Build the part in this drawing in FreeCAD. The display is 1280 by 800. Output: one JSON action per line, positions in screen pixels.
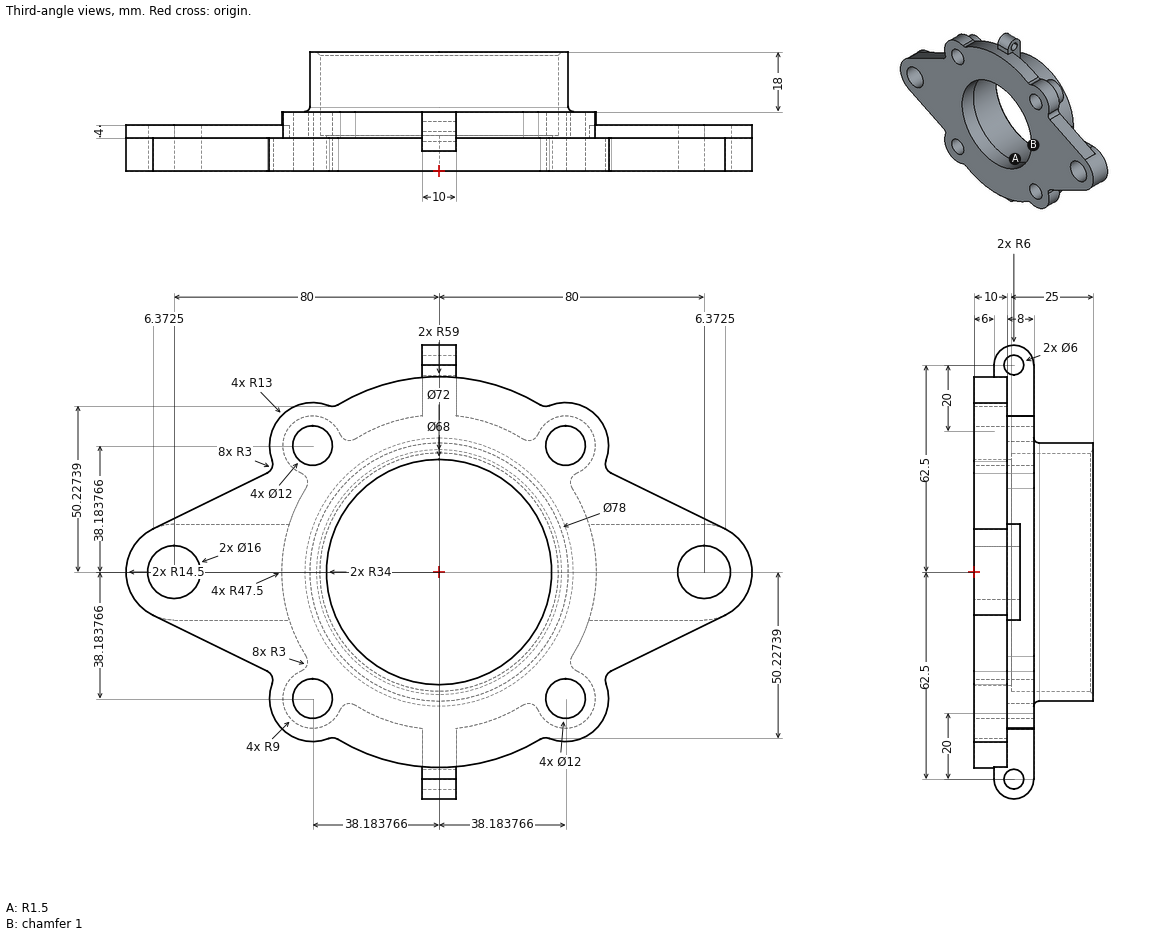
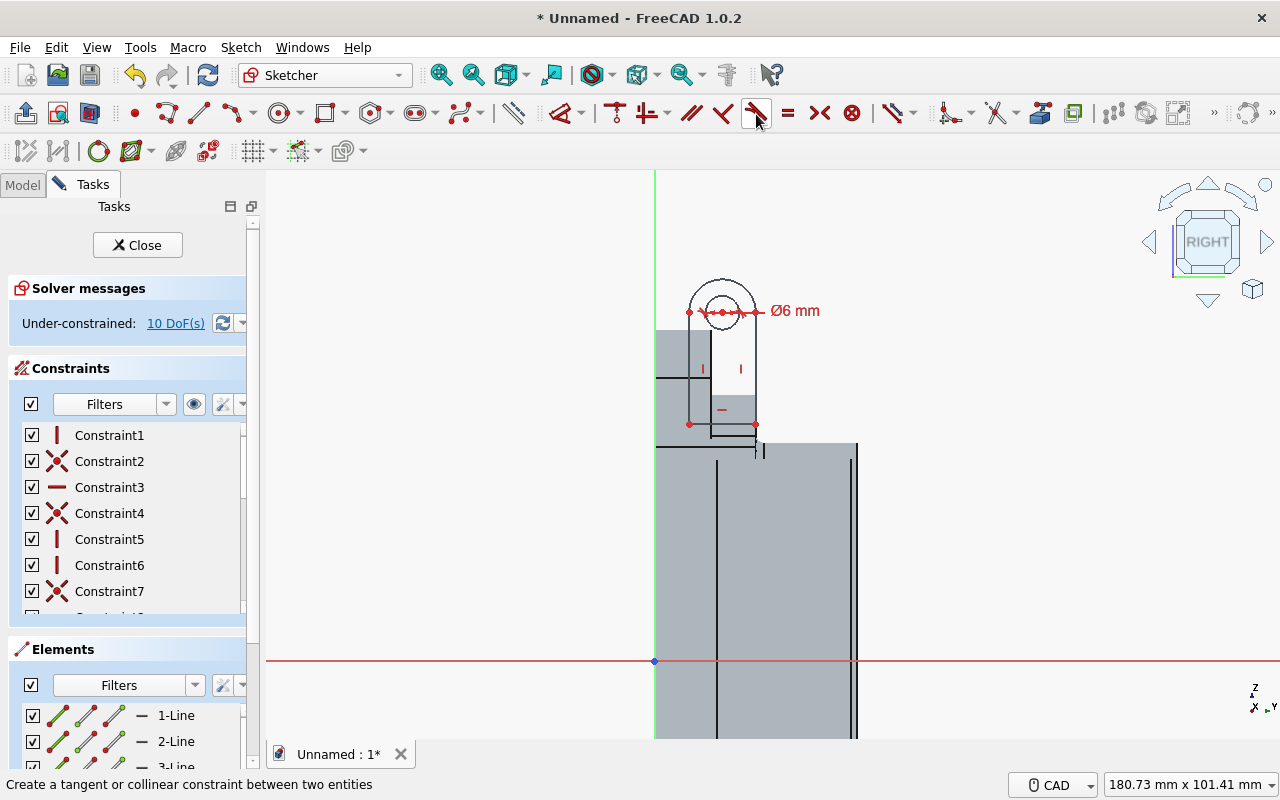
{"action": "scroll", "coordinate": [704, 286], "scroll_direction": "down", "scroll_amount": 4}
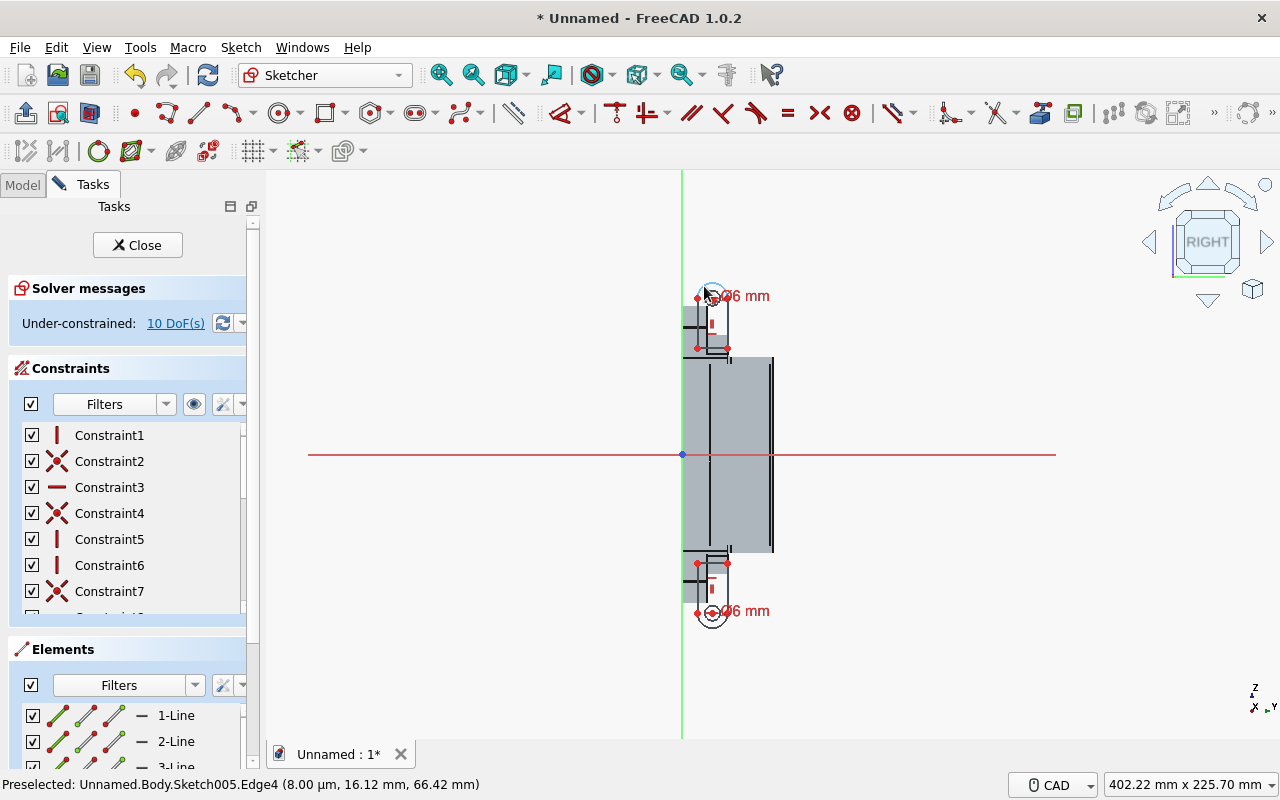
{"action": "left_click", "coordinate": [728, 598]}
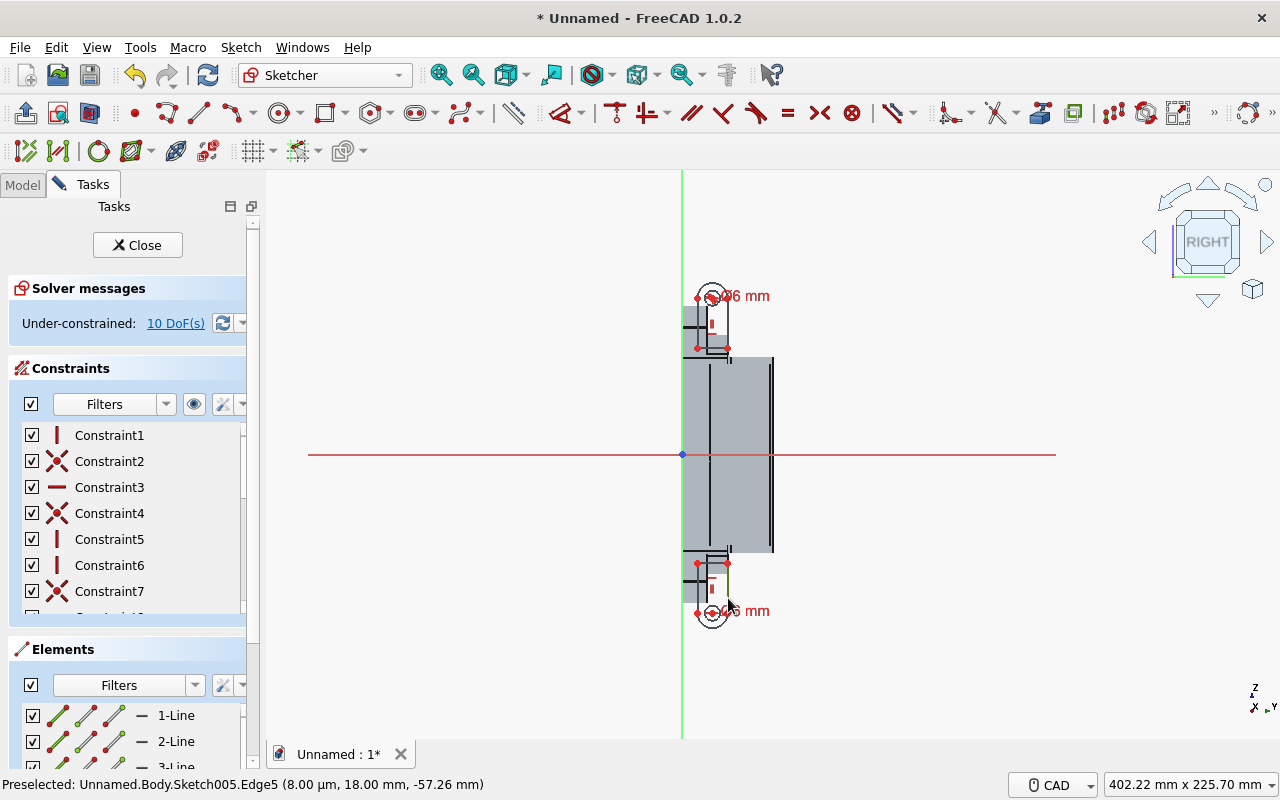
{"action": "scroll", "coordinate": [713, 628], "scroll_direction": "up", "scroll_amount": 4}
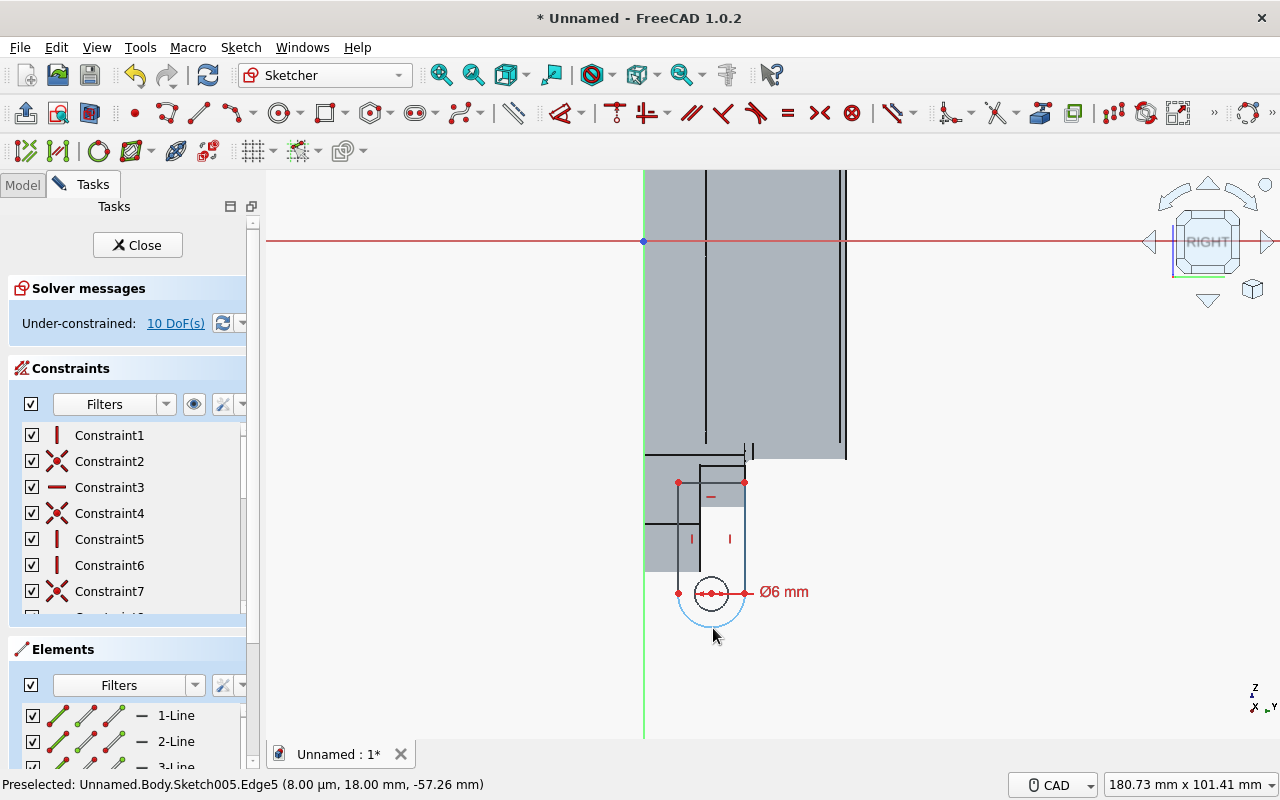
{"action": "left_click", "coordinate": [711, 627]}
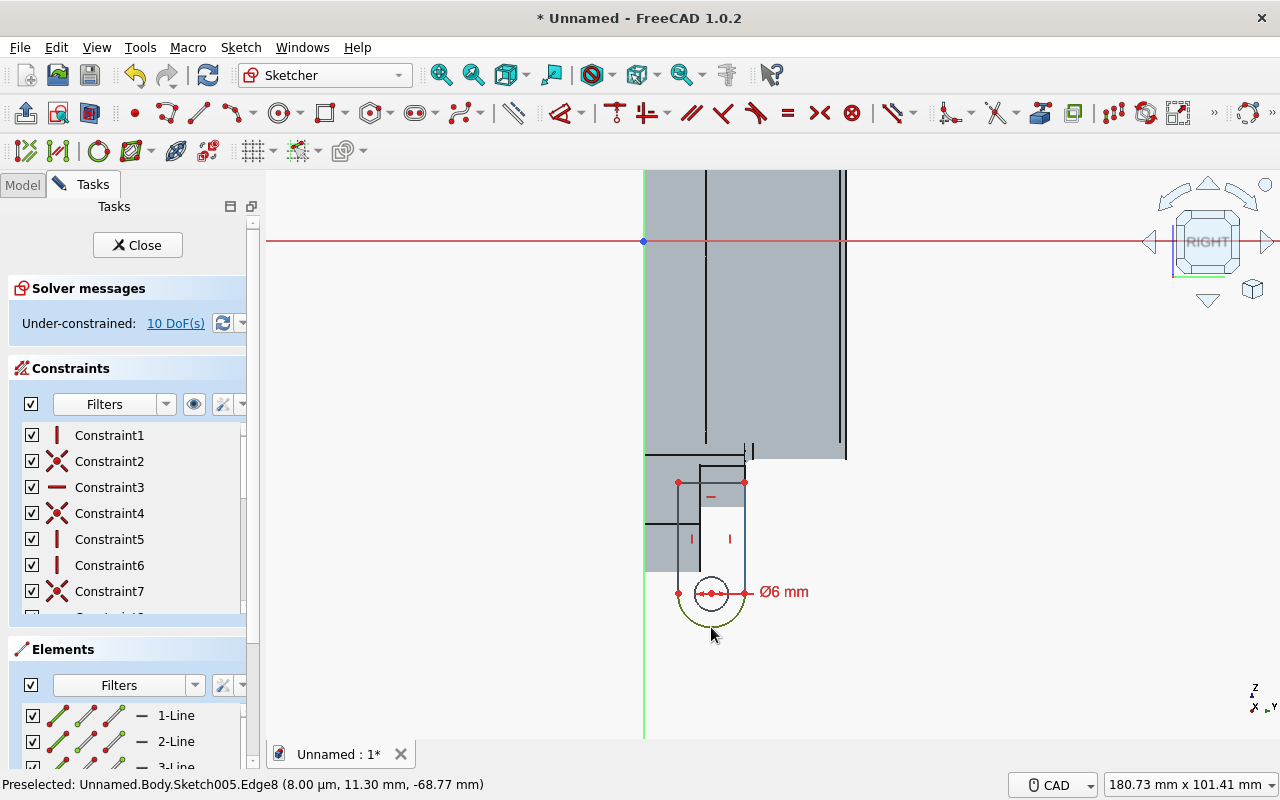
{"action": "left_click", "coordinate": [756, 114]}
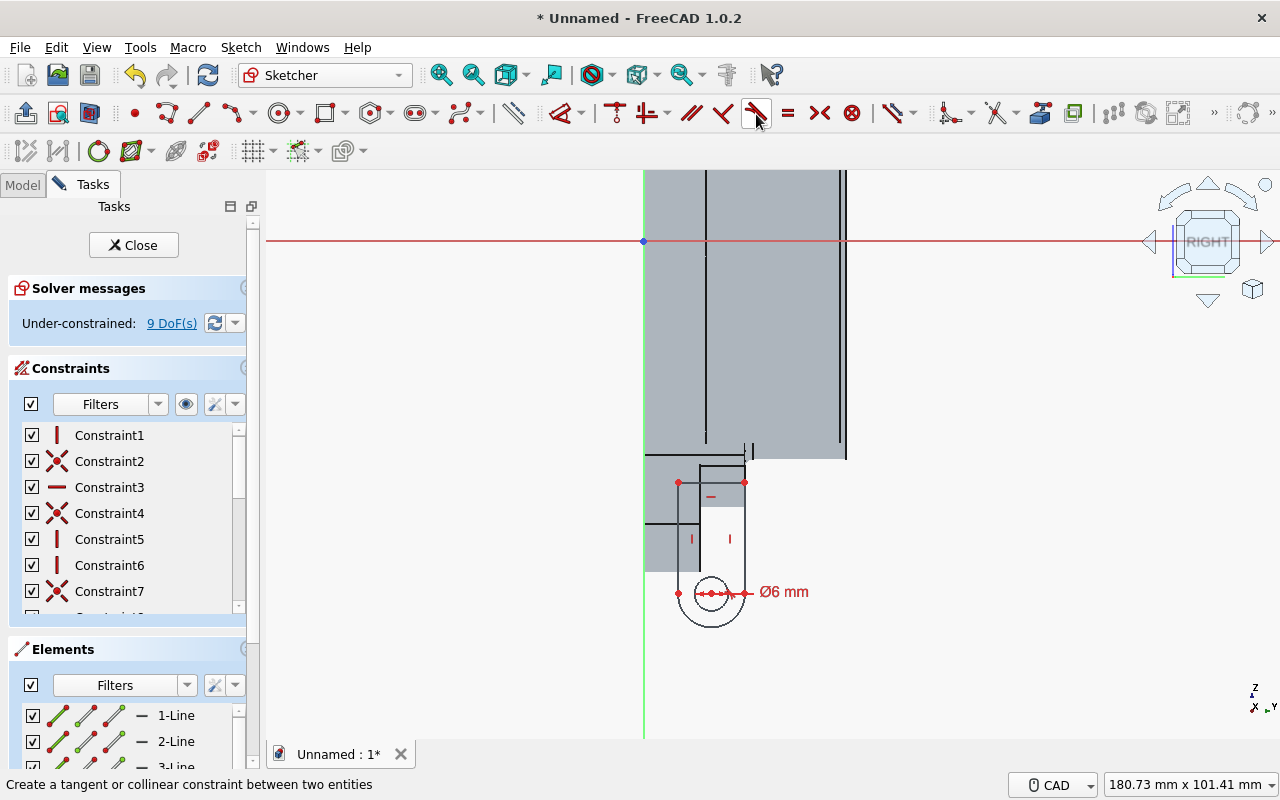
{"action": "left_click", "coordinate": [678, 516]}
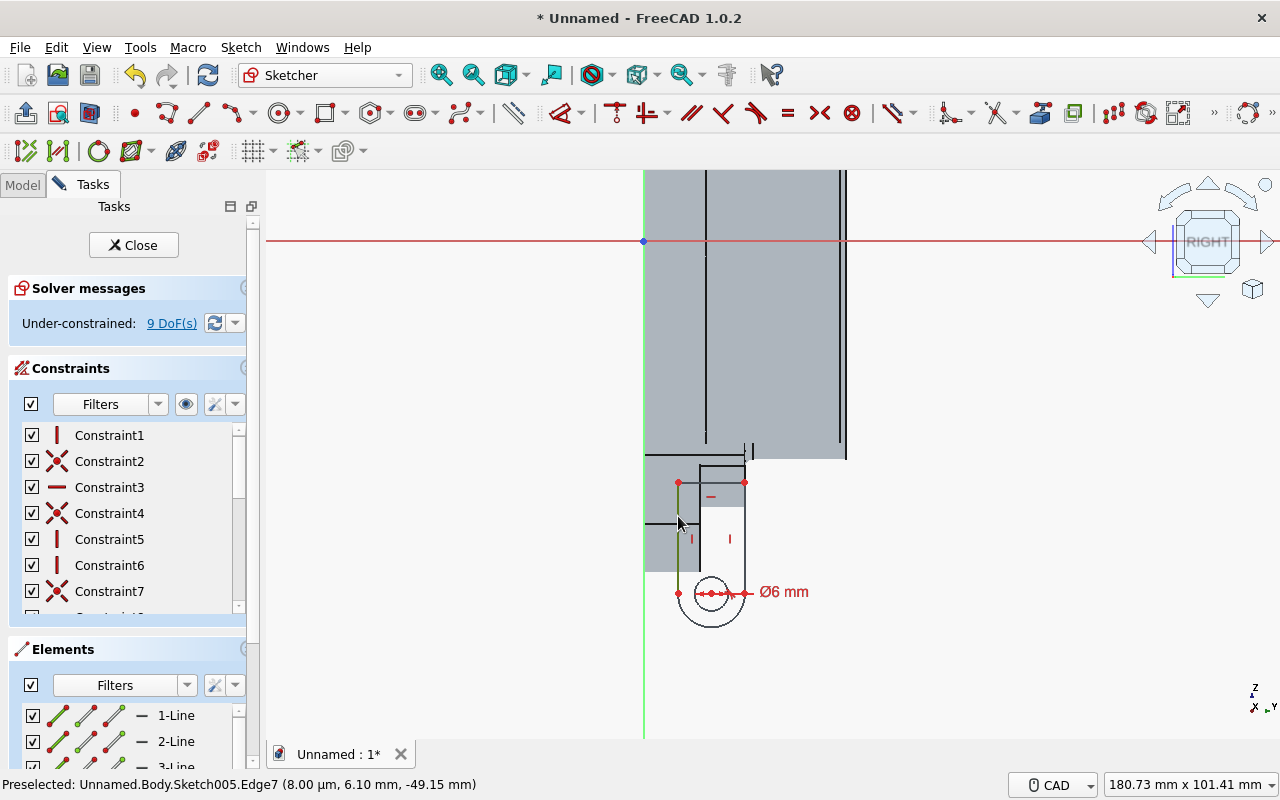
{"action": "left_click", "coordinate": [692, 621]}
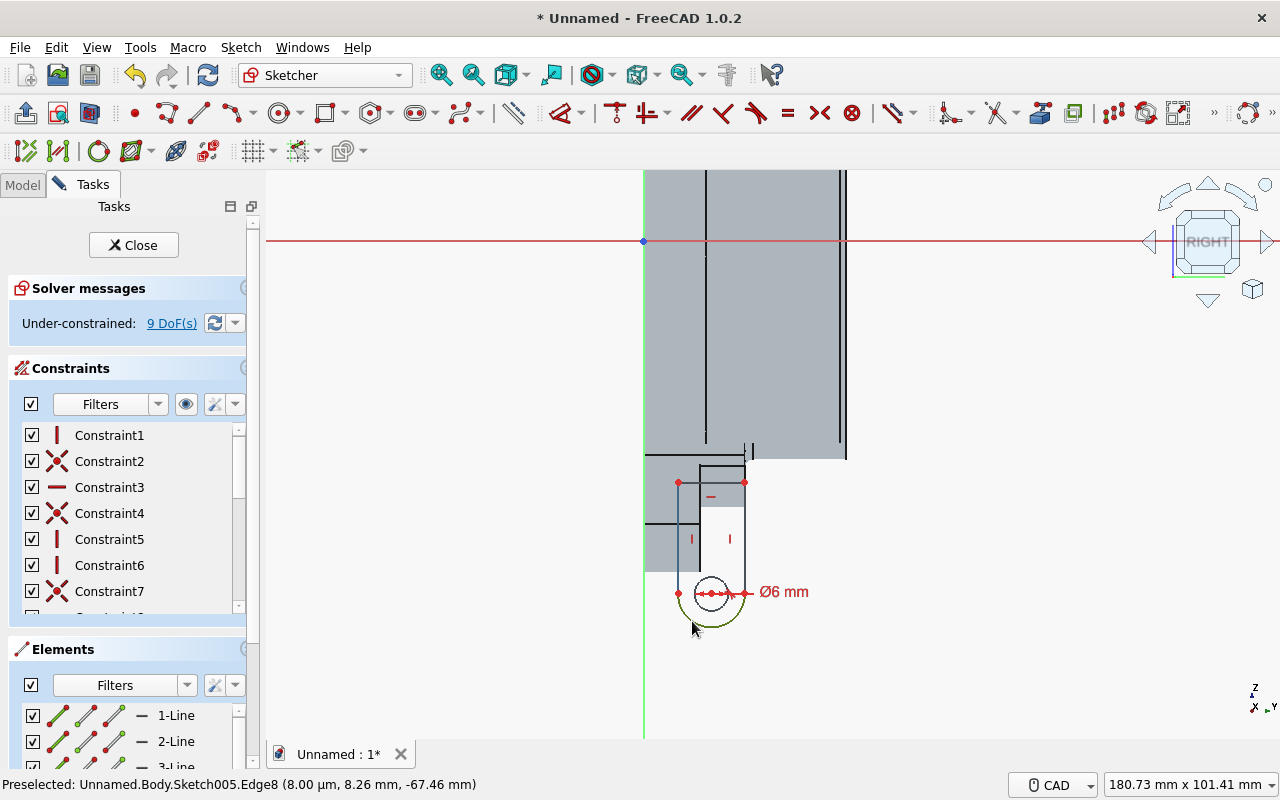
{"action": "left_click", "coordinate": [756, 114]}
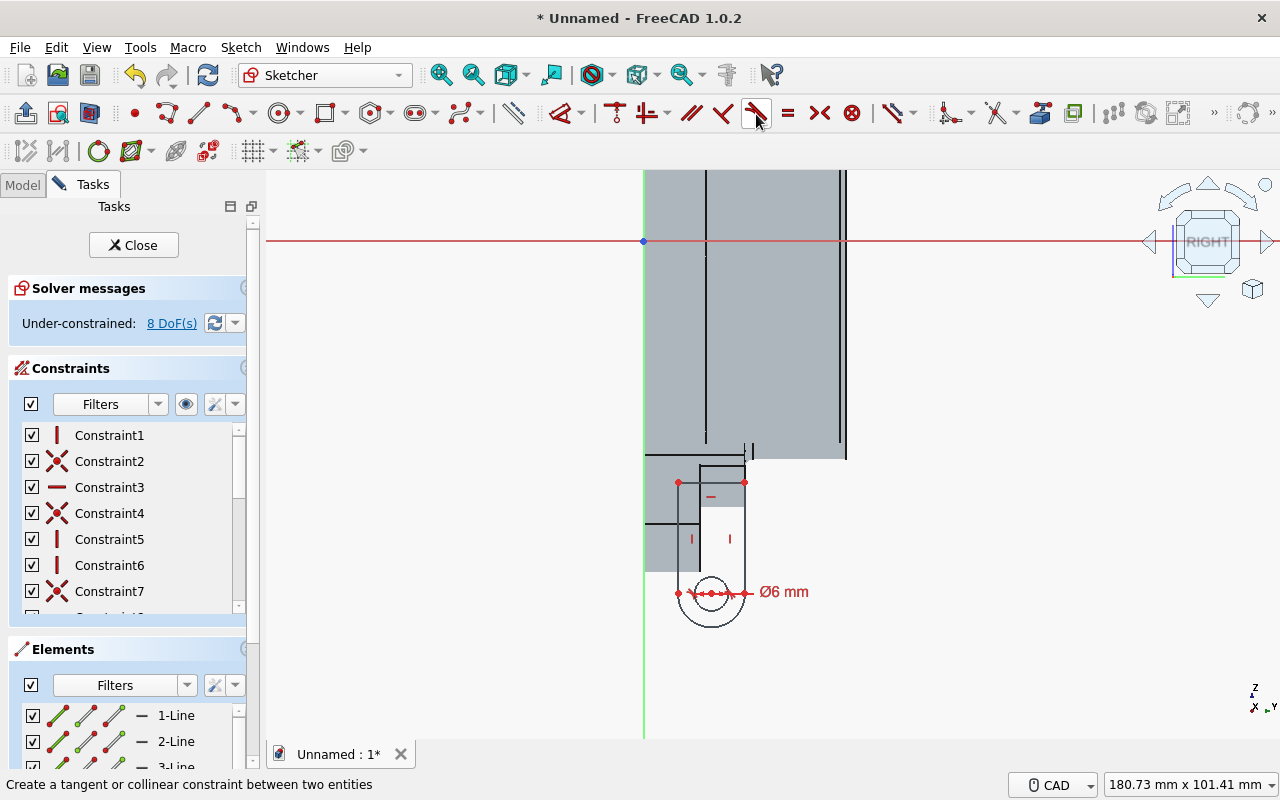
{"action": "scroll", "coordinate": [713, 629], "scroll_direction": "down", "scroll_amount": 4}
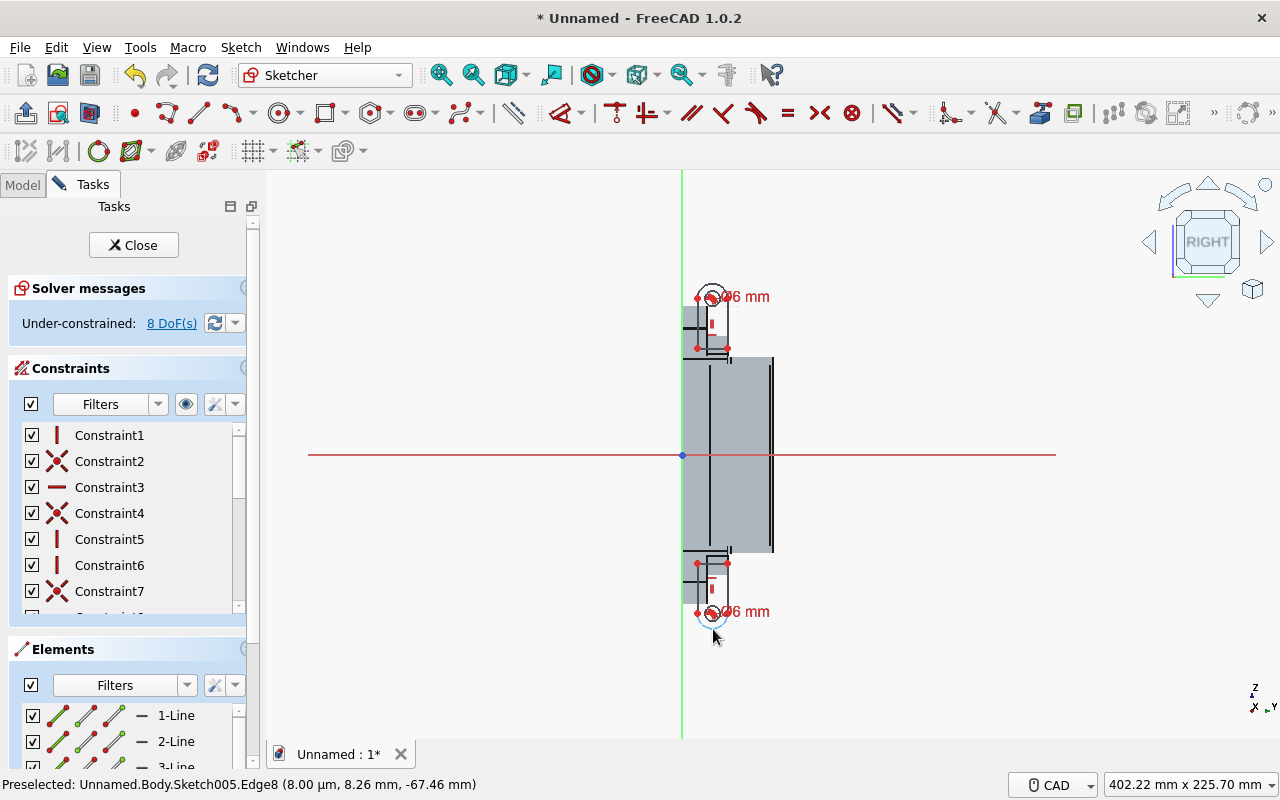
{"action": "scroll", "coordinate": [721, 287], "scroll_direction": "up", "scroll_amount": 4}